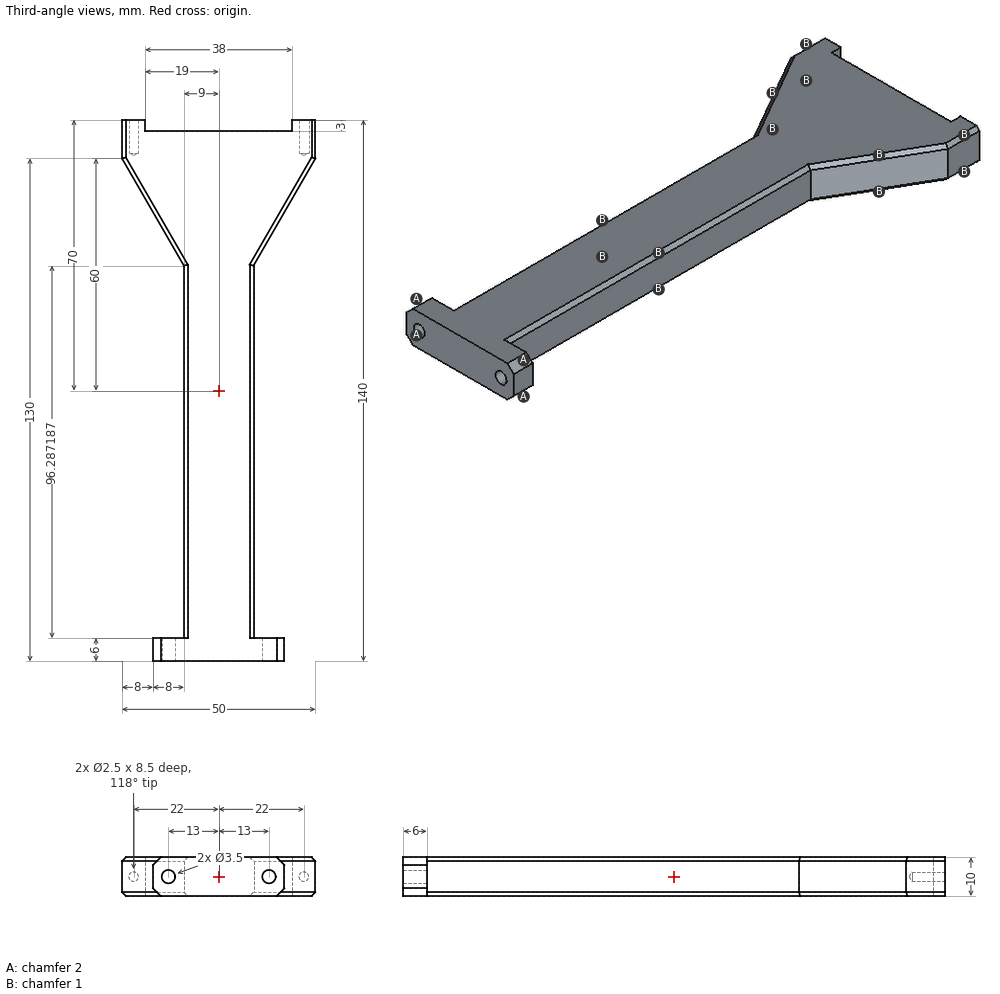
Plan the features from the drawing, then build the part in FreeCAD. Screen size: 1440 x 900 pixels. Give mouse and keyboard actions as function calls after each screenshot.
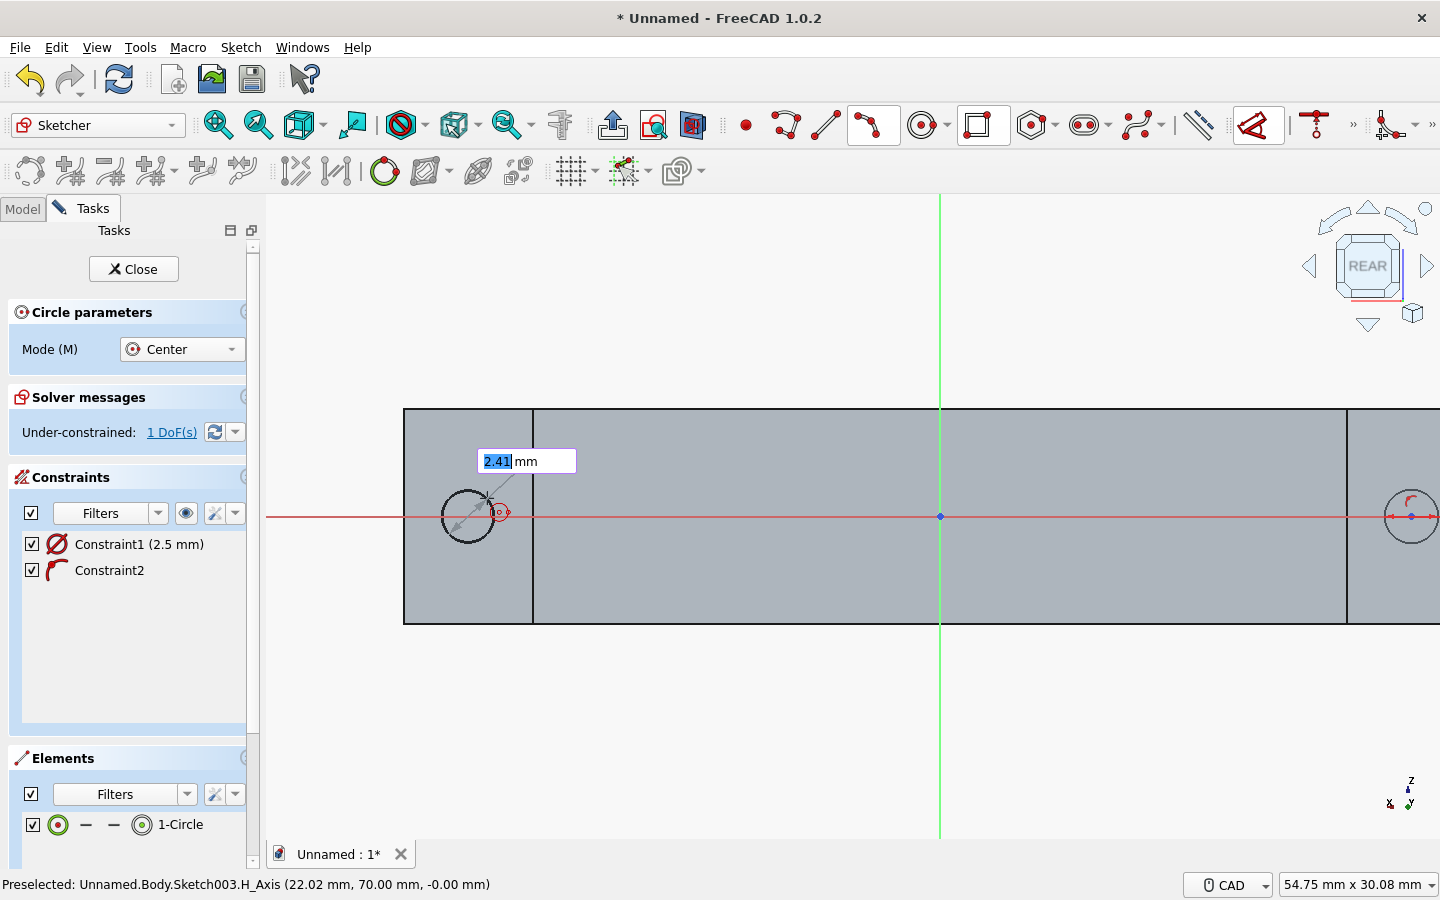
text(2.5)
key(Return)
key(Escape)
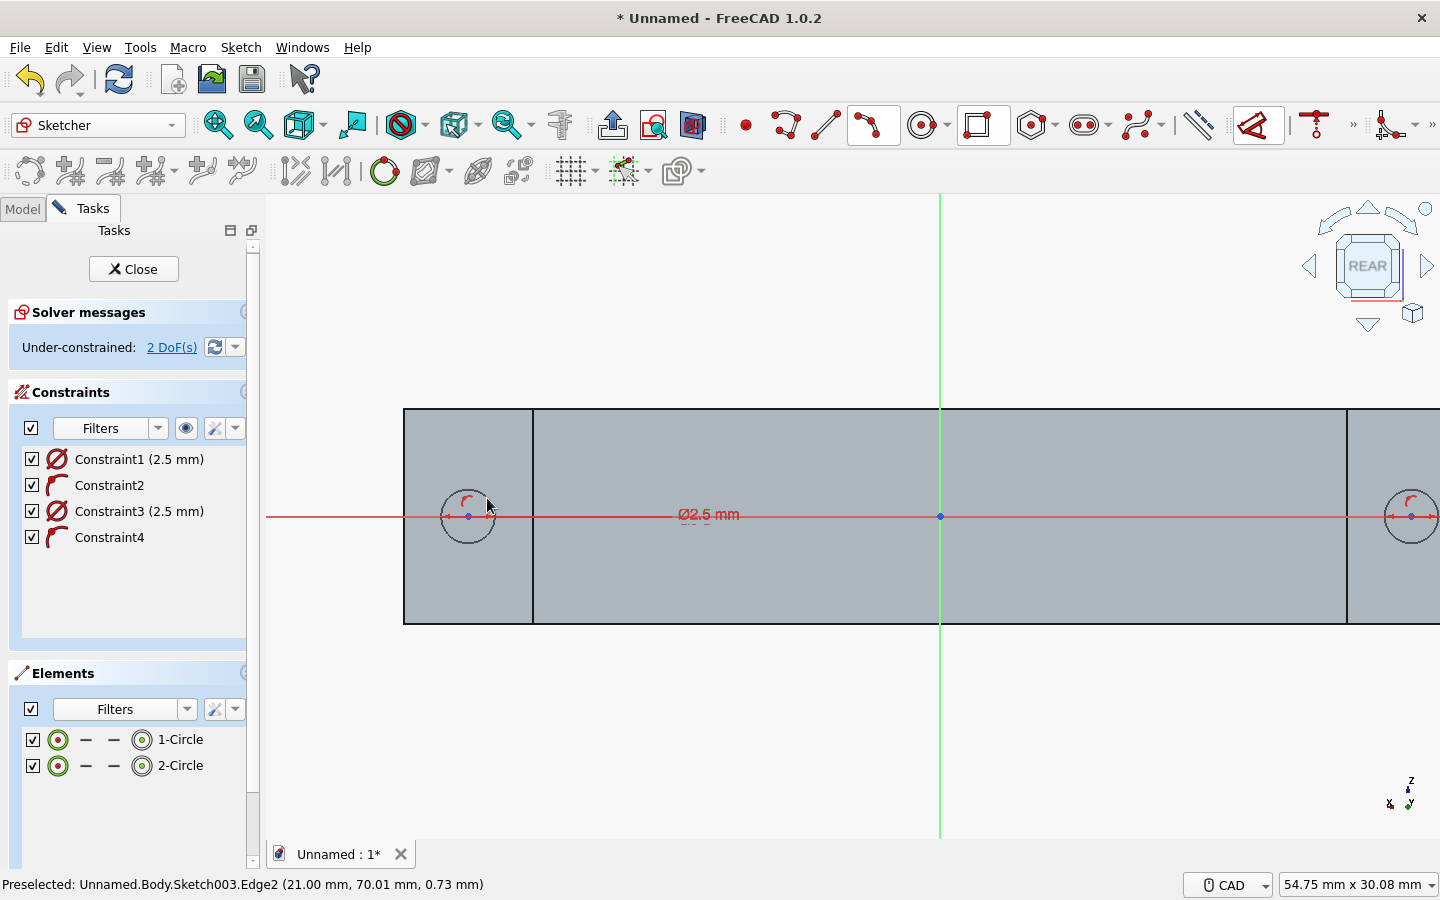
scroll(468, 516, down, 2)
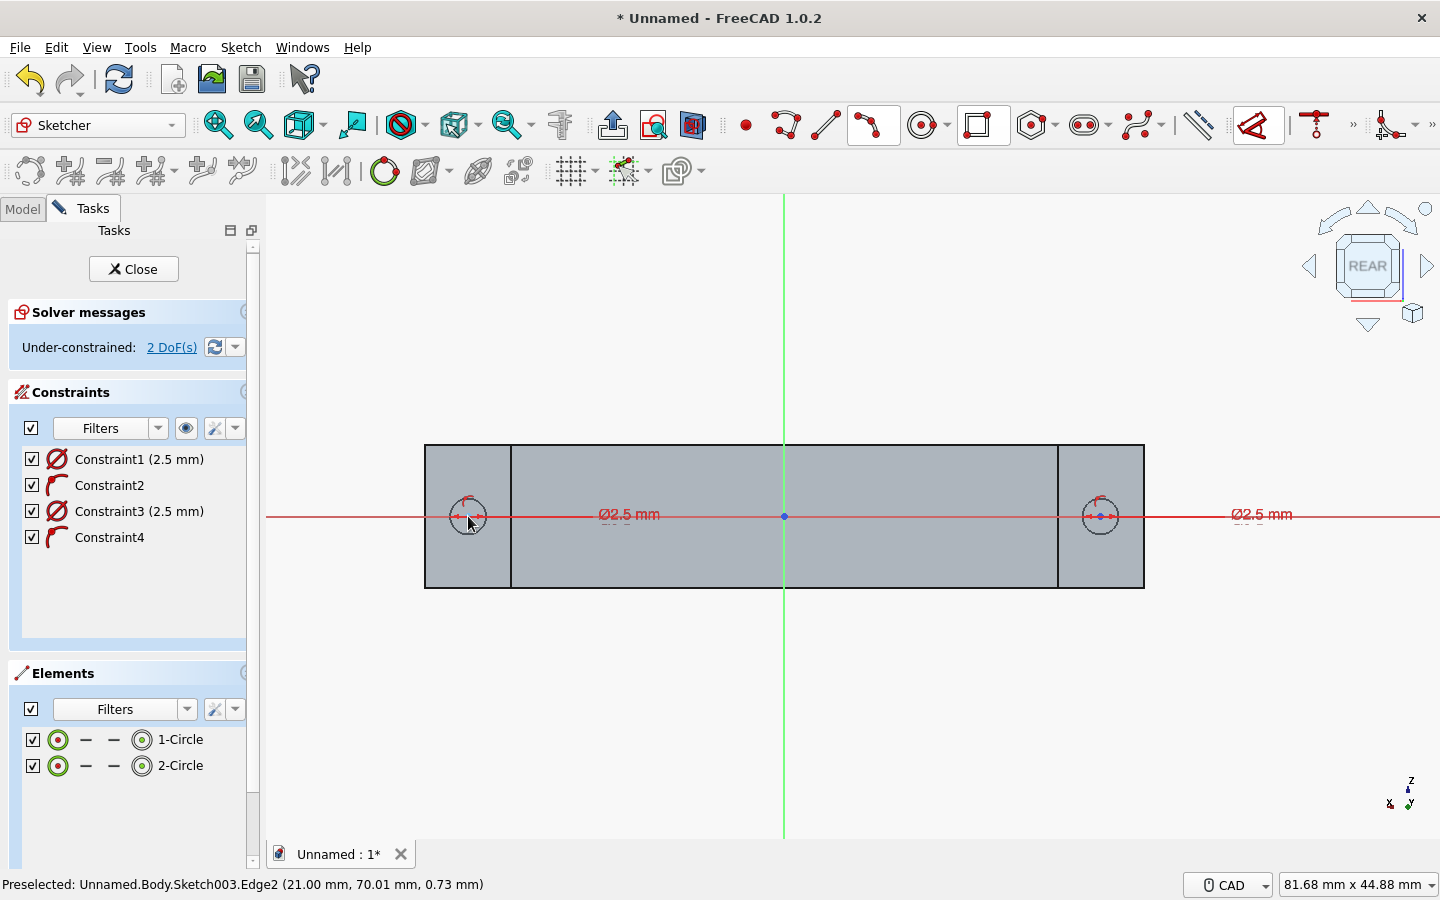
click(1101, 516)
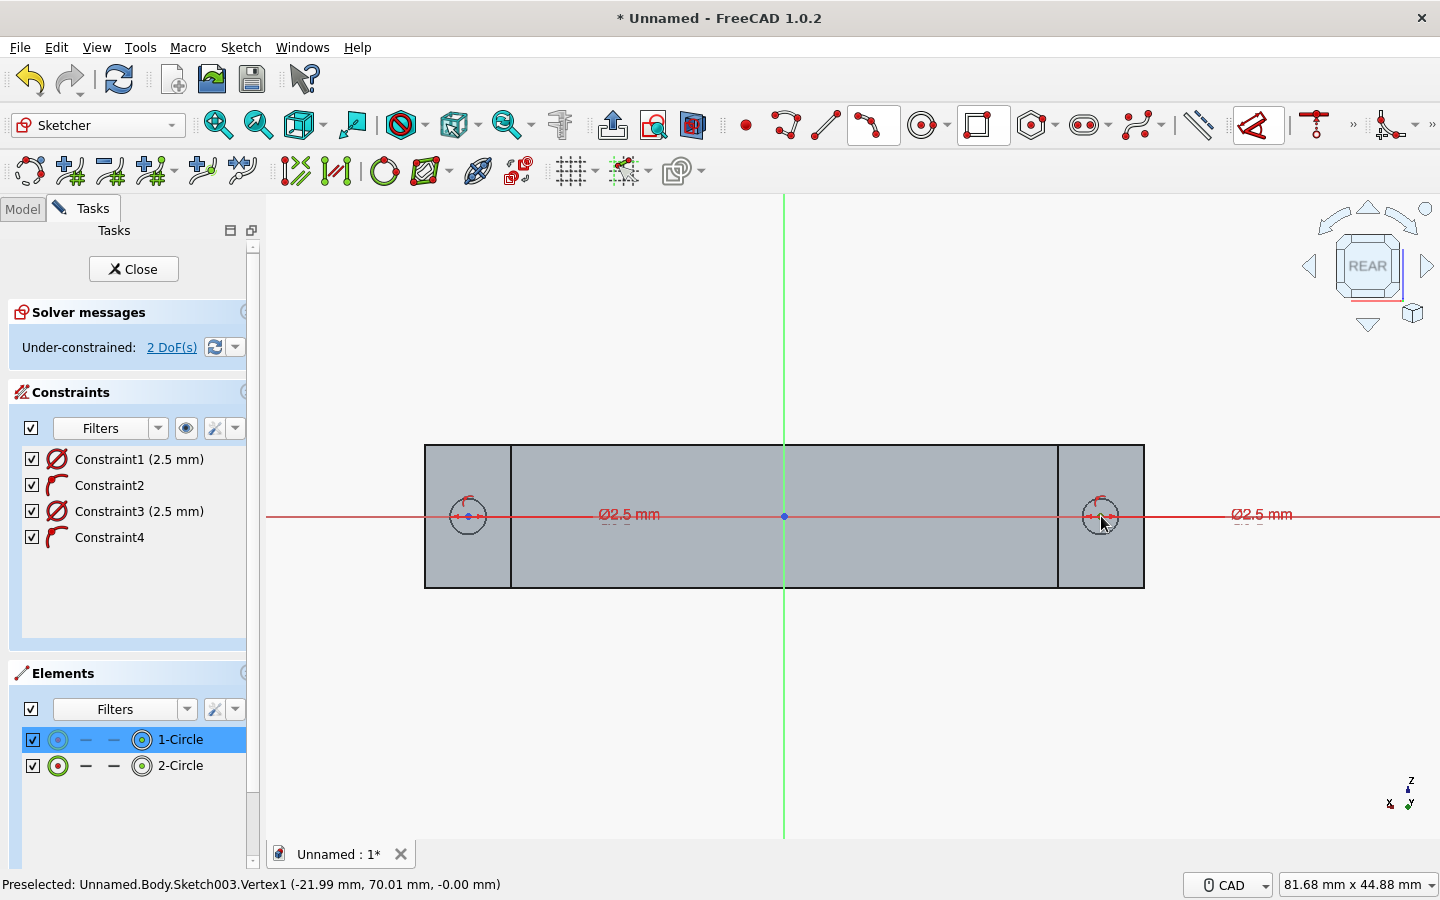
click(1278, 126)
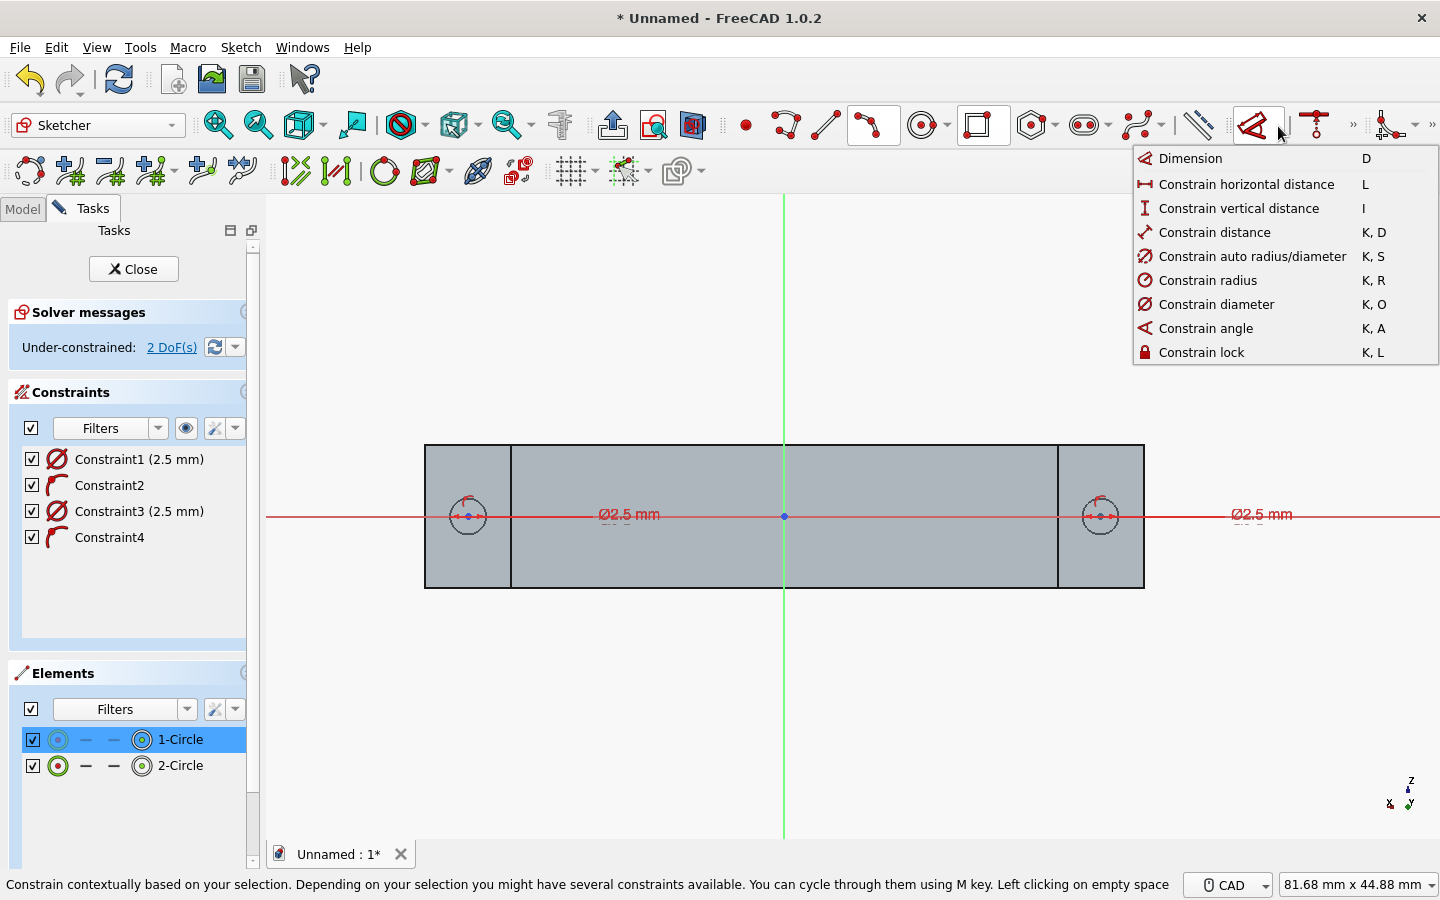
click(1286, 184)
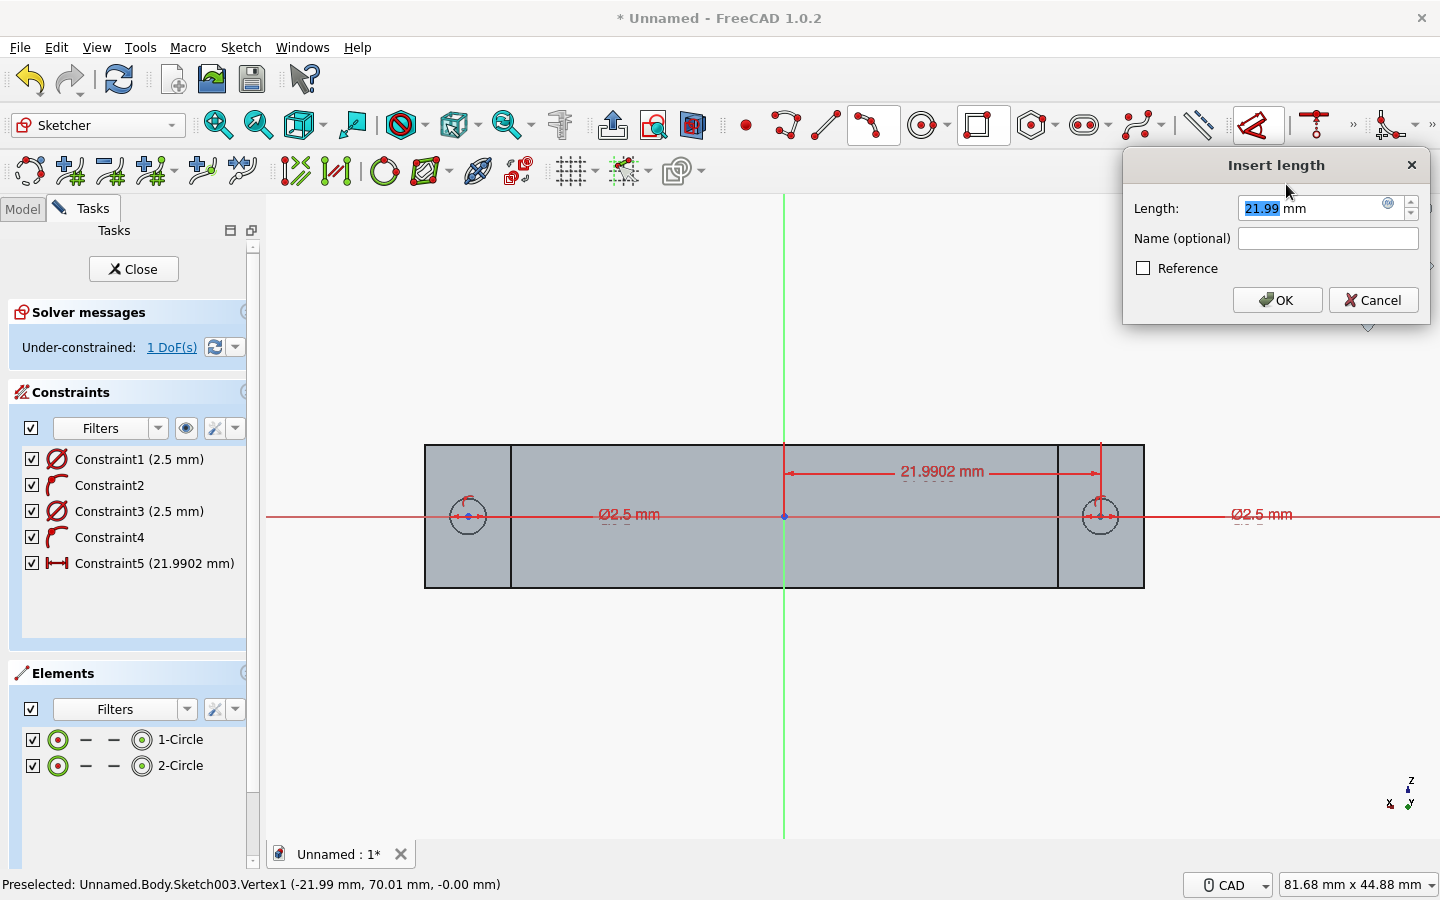
text(22)
key(Return)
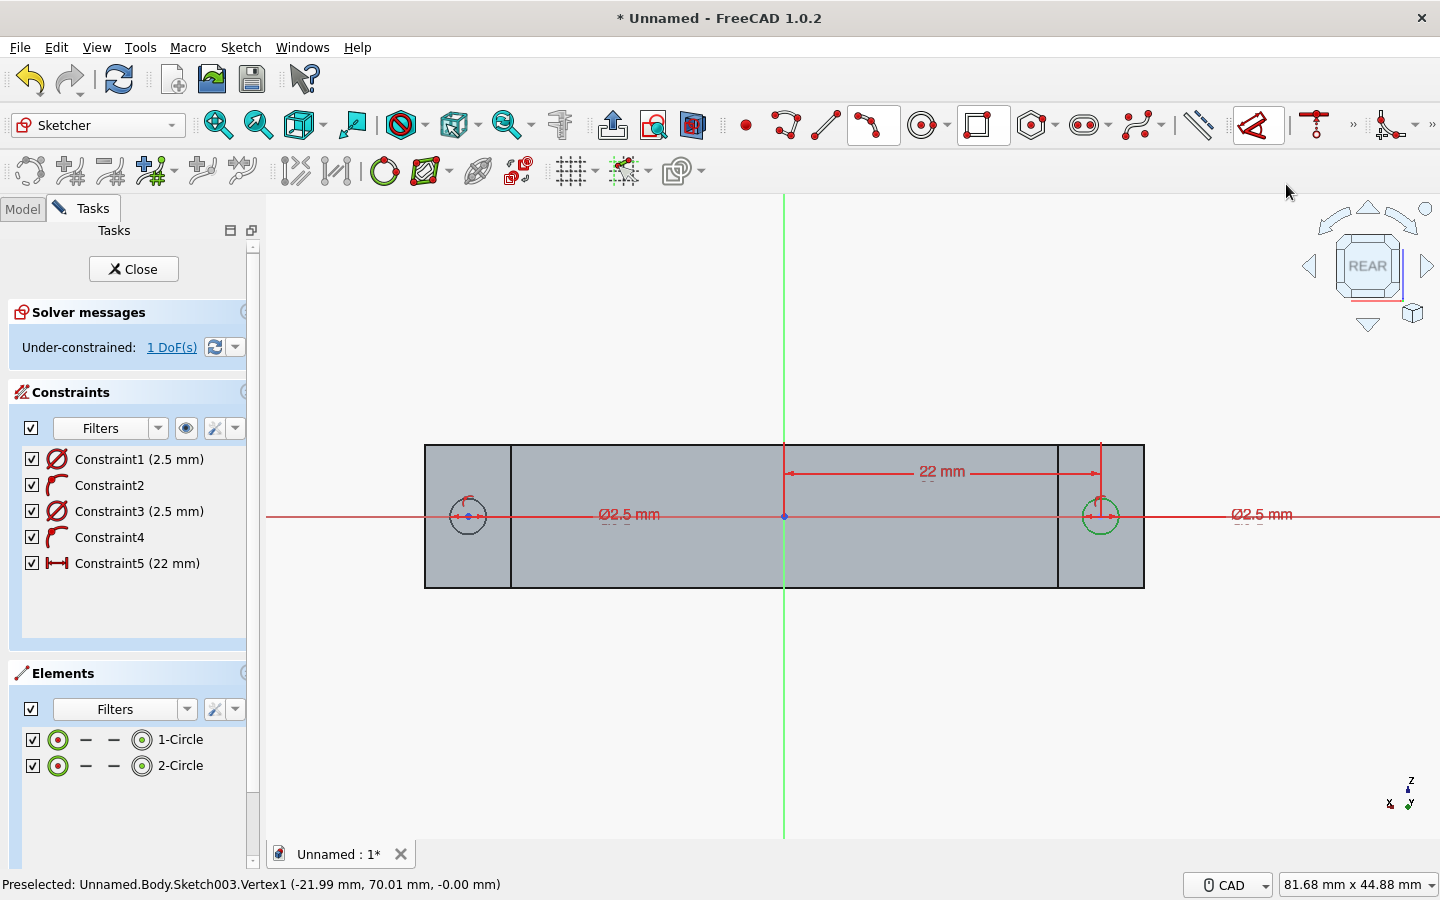
click(468, 516)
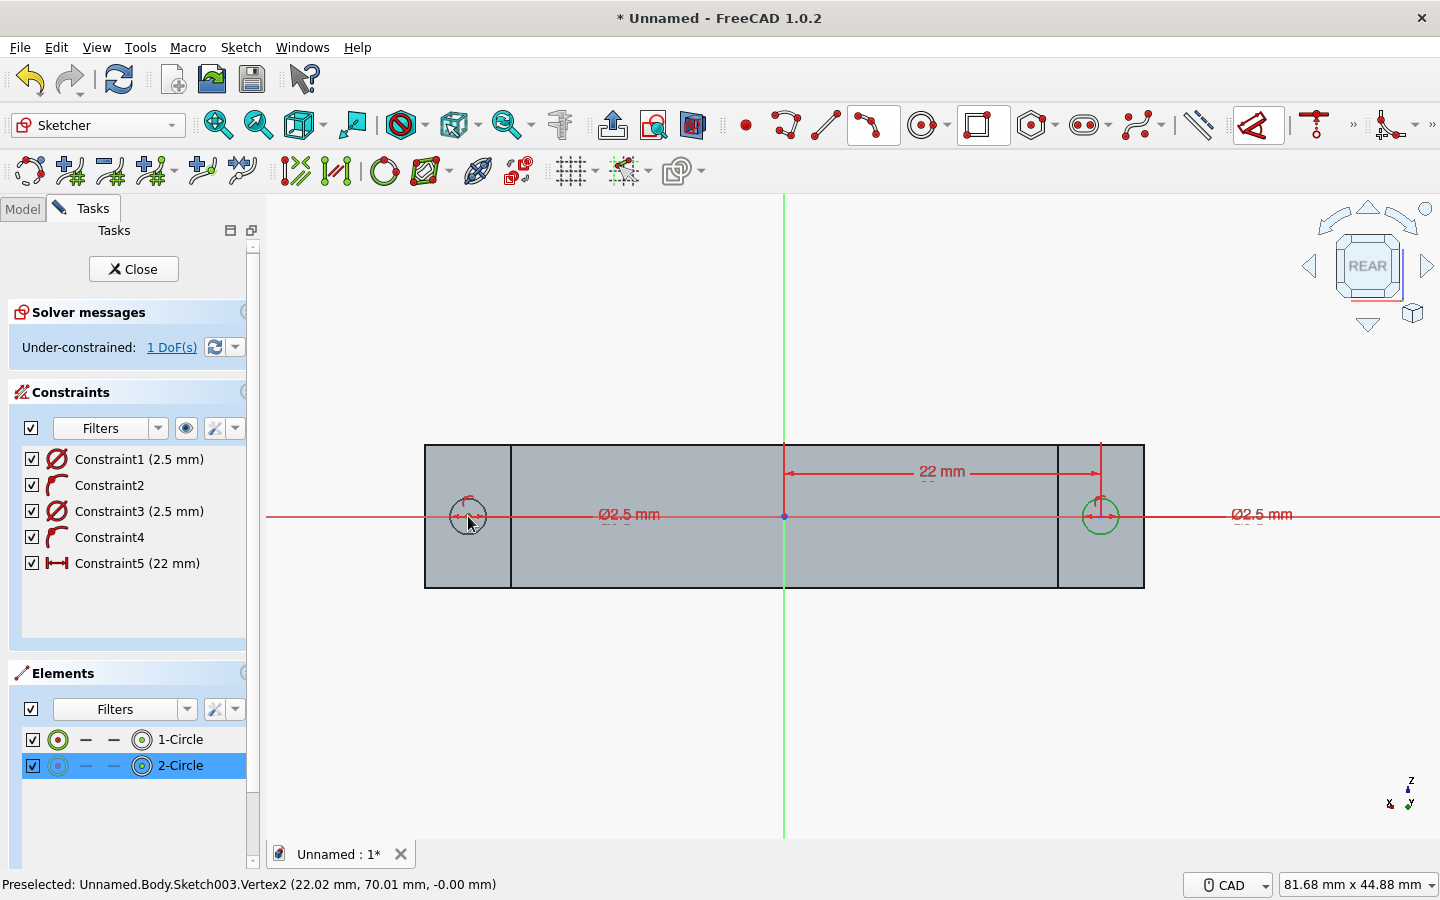
click(1278, 126)